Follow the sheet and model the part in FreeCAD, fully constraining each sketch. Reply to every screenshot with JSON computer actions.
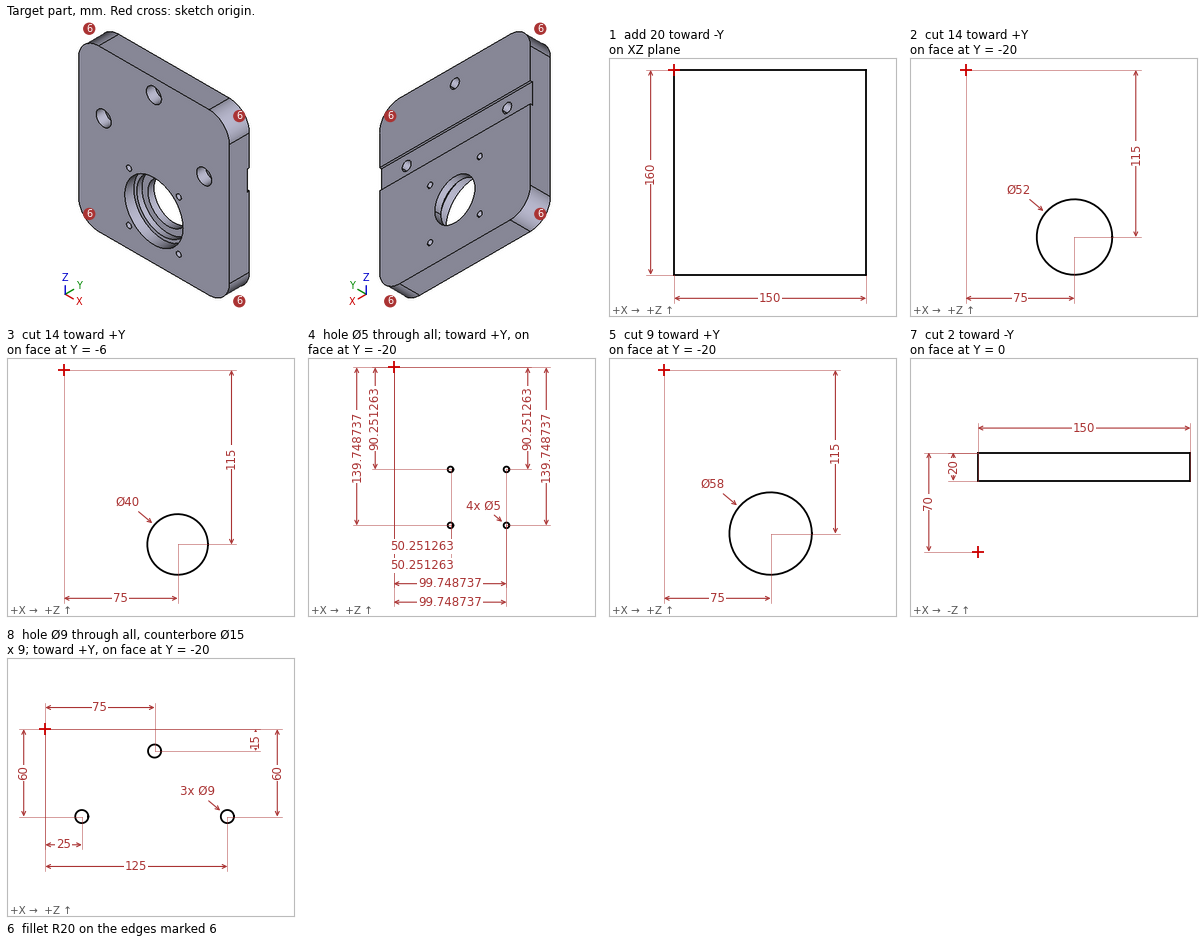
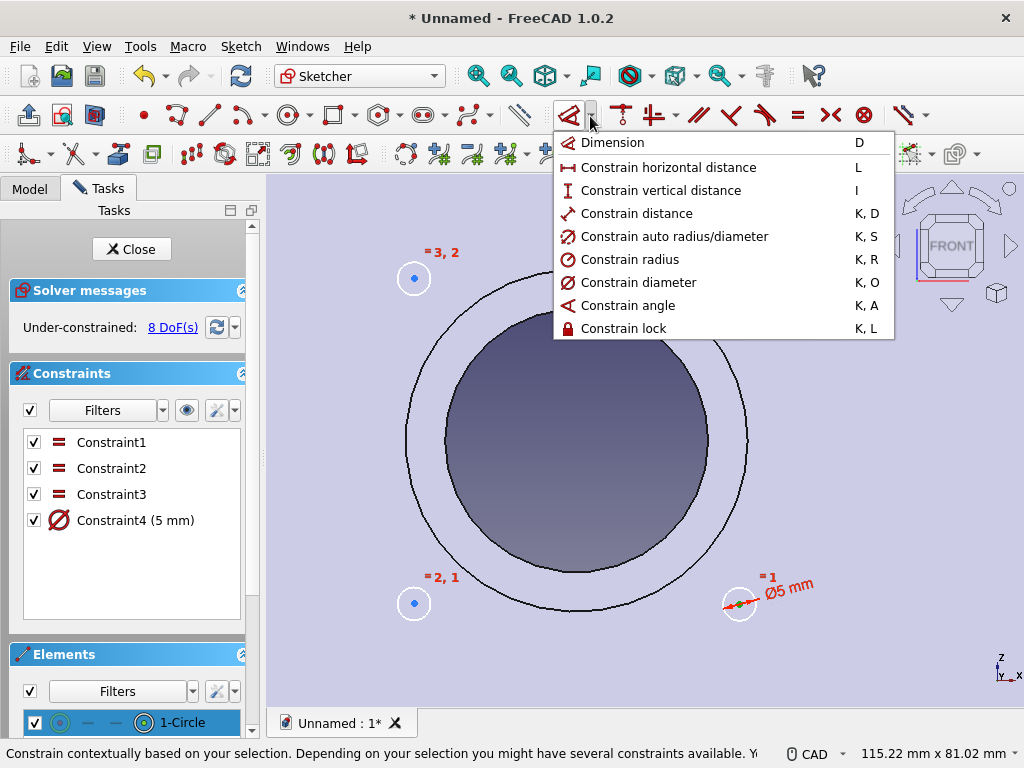
{"action": "left_click", "coordinate": [724, 168]}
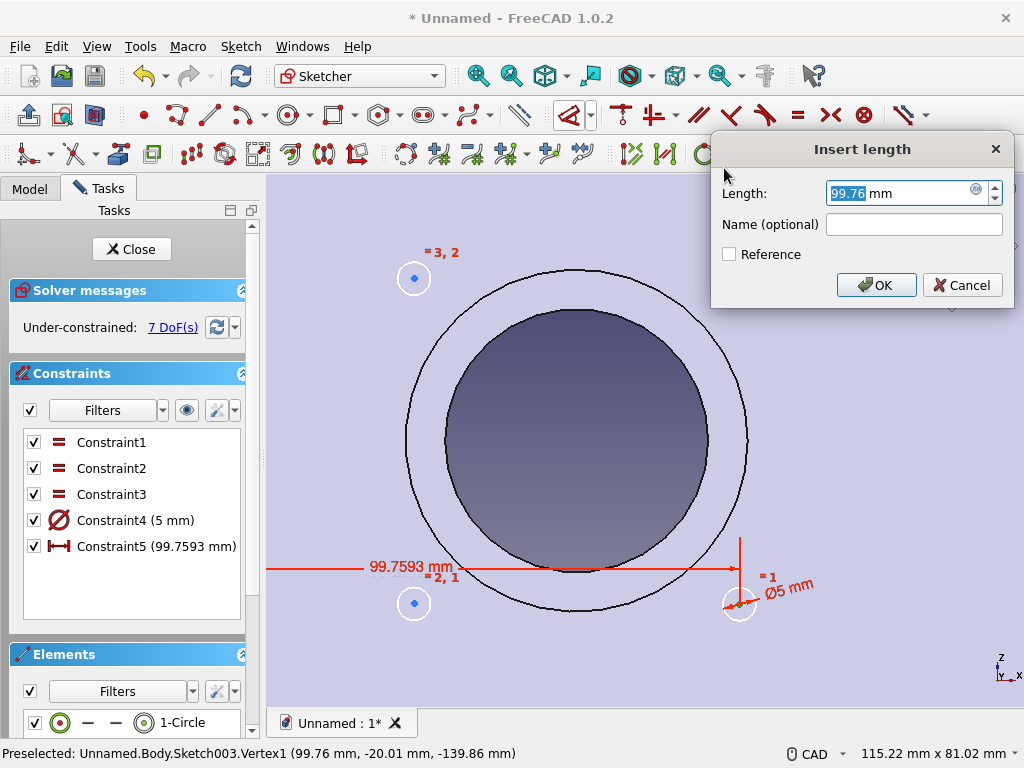
{"action": "type", "text": "99.748737"}
{"action": "key", "text": "Return"}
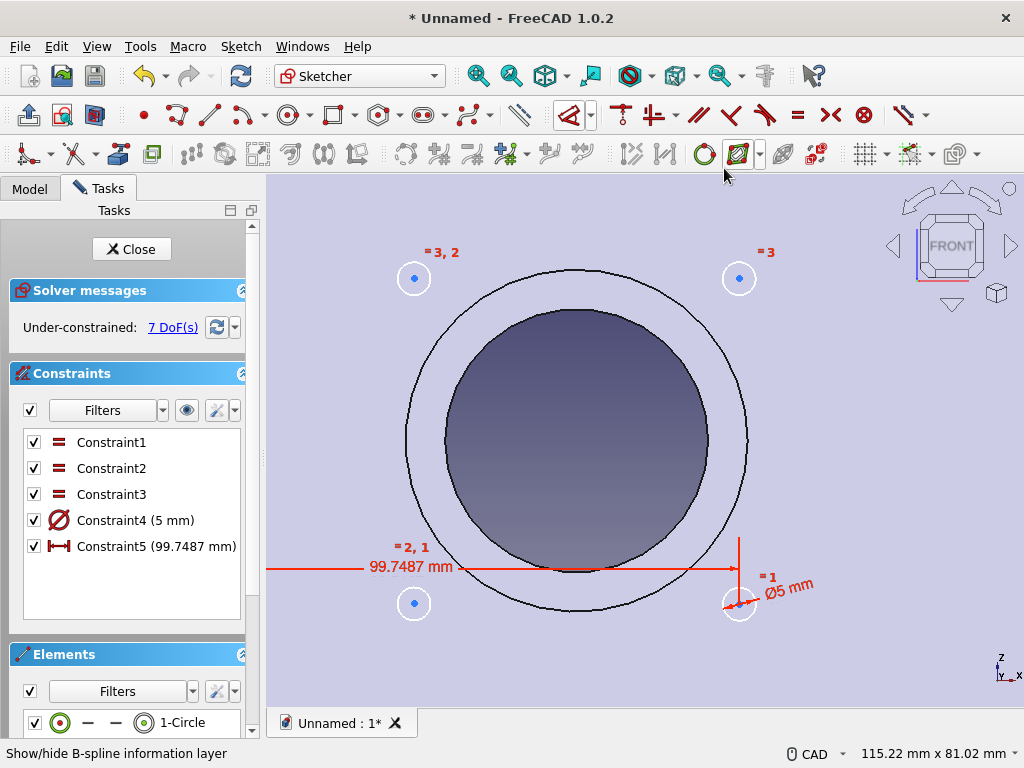
{"action": "left_click", "coordinate": [414, 604]}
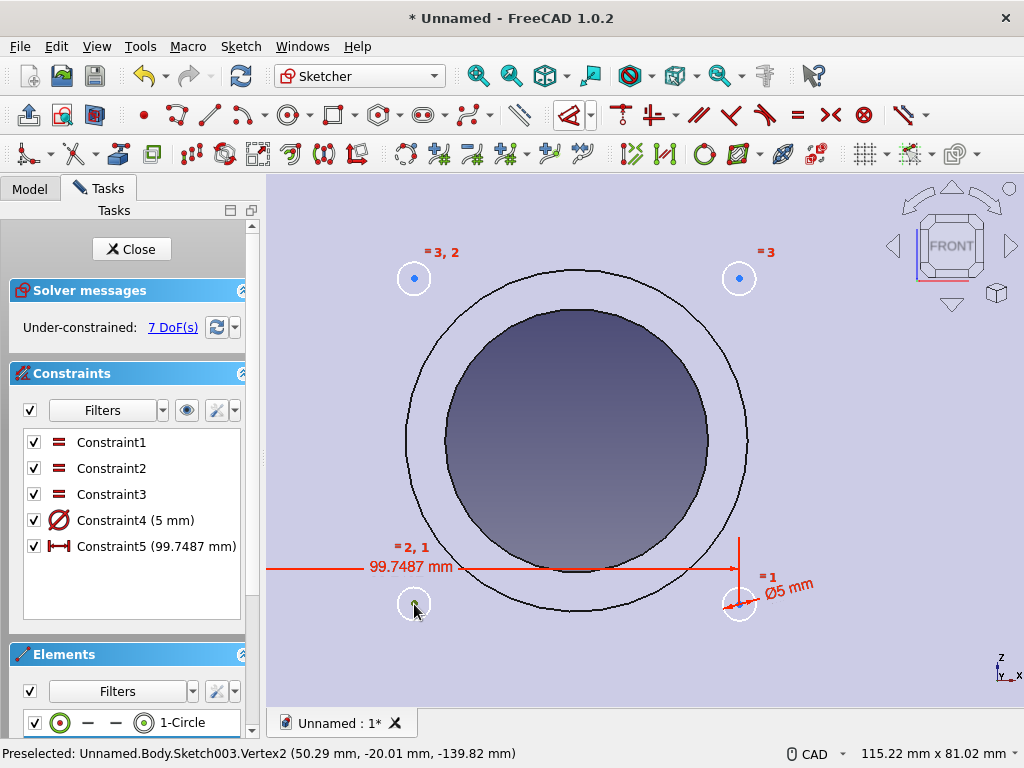
{"action": "key", "text": "l"}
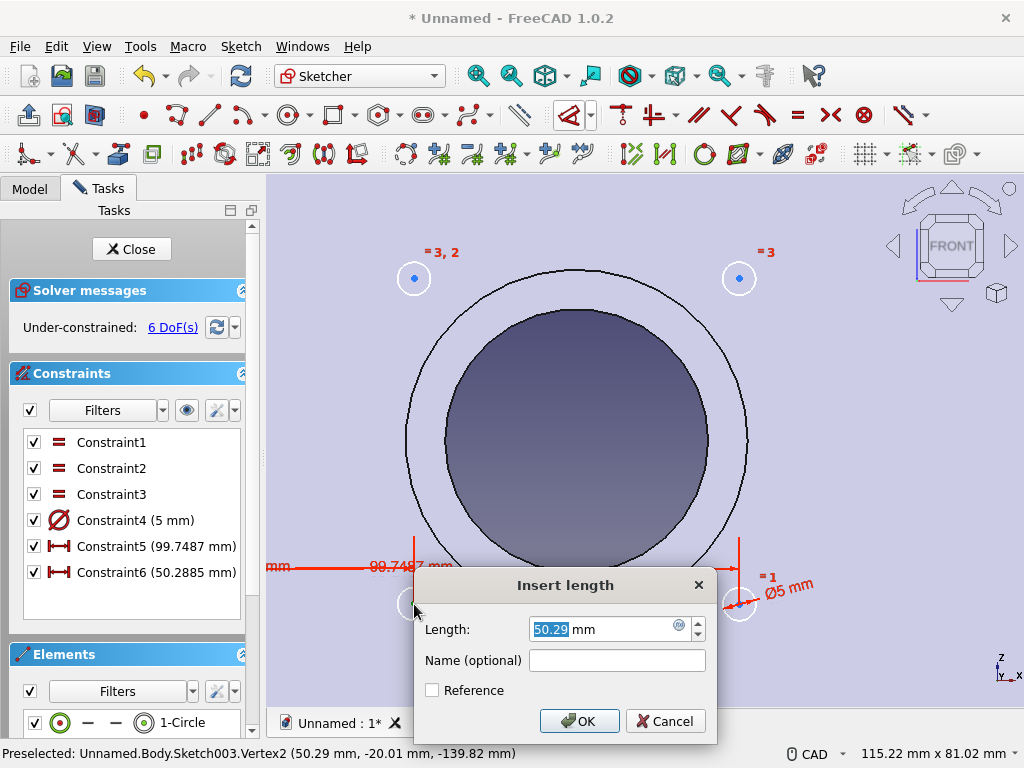
{"action": "type", "text": "50.251263"}
{"action": "key", "text": "Return"}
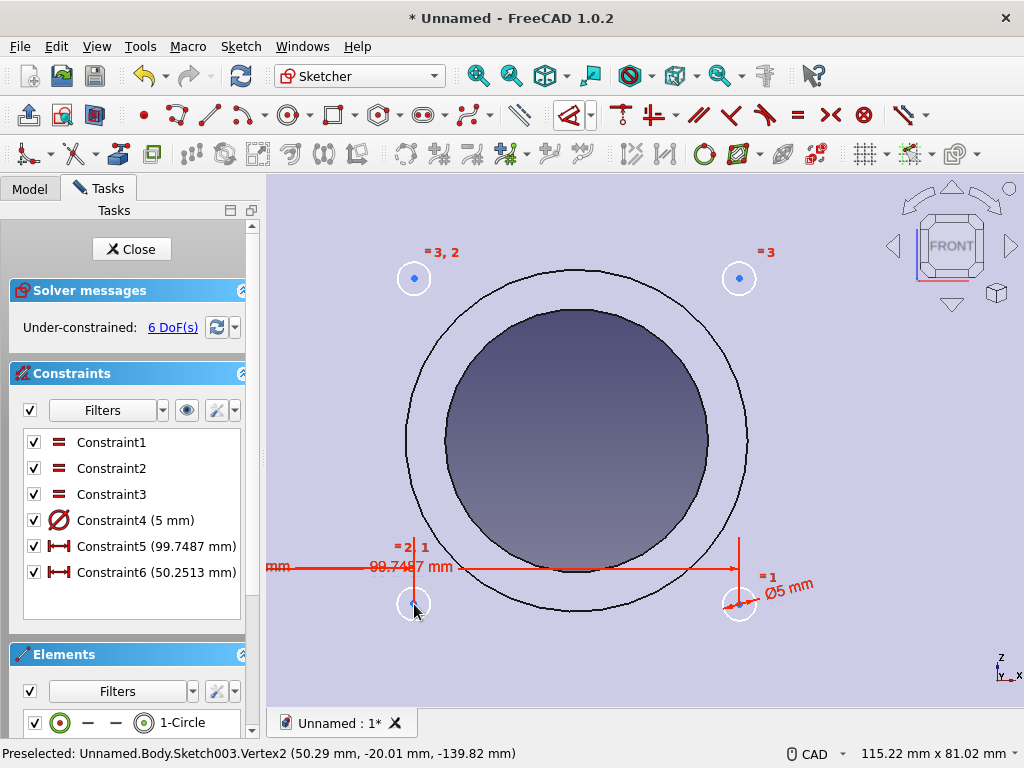
{"action": "left_click", "coordinate": [414, 279]}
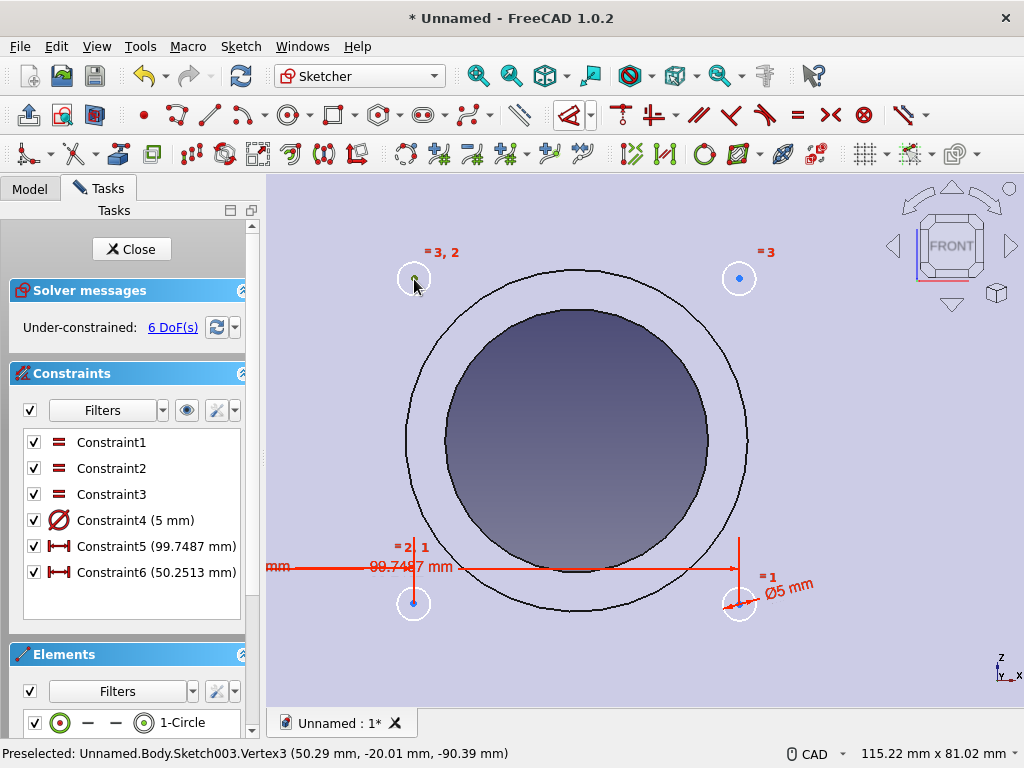
{"action": "key", "text": "l"}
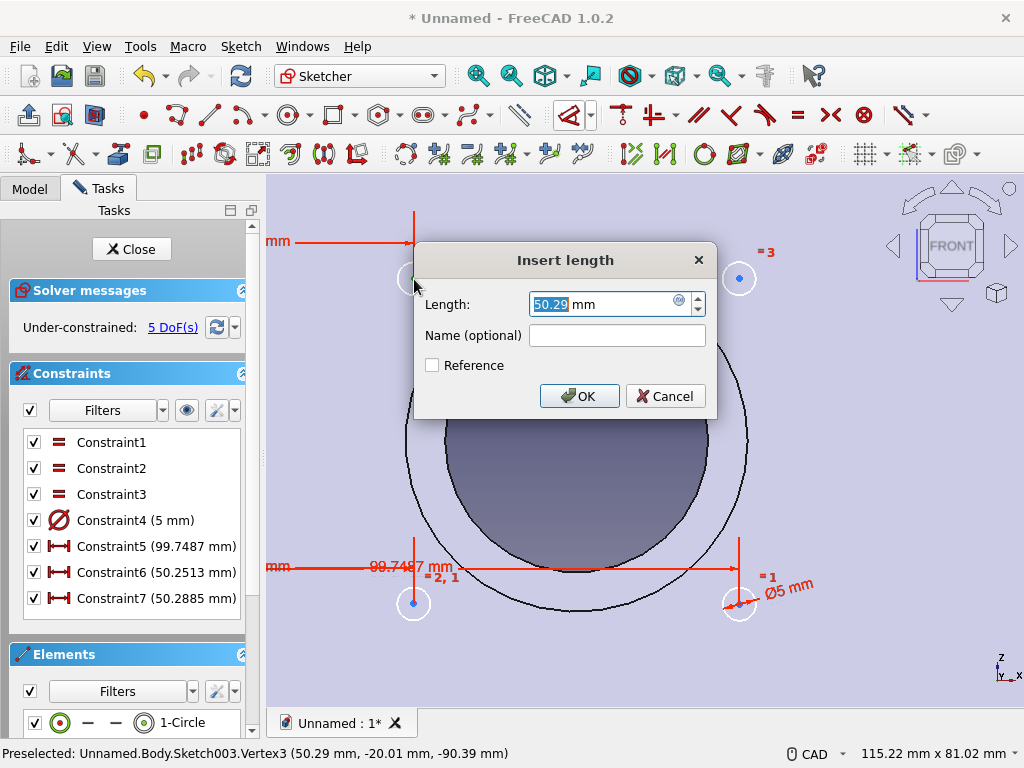
{"action": "type", "text": "50.251263"}
{"action": "key", "text": "Return"}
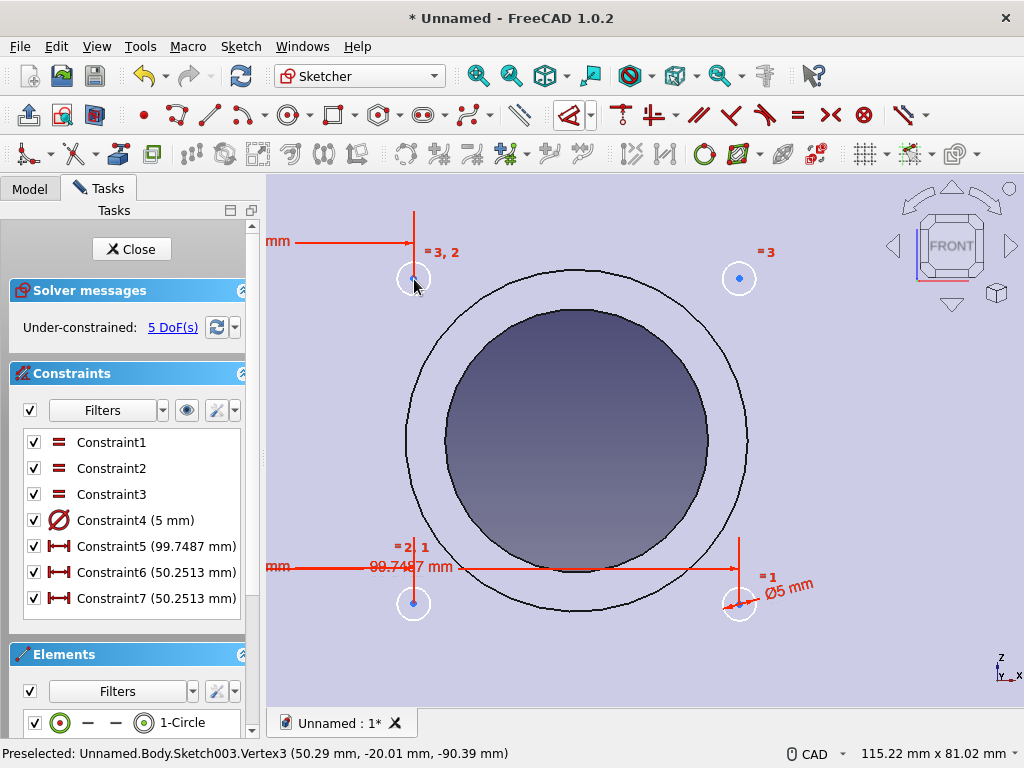
{"action": "left_click", "coordinate": [414, 279]}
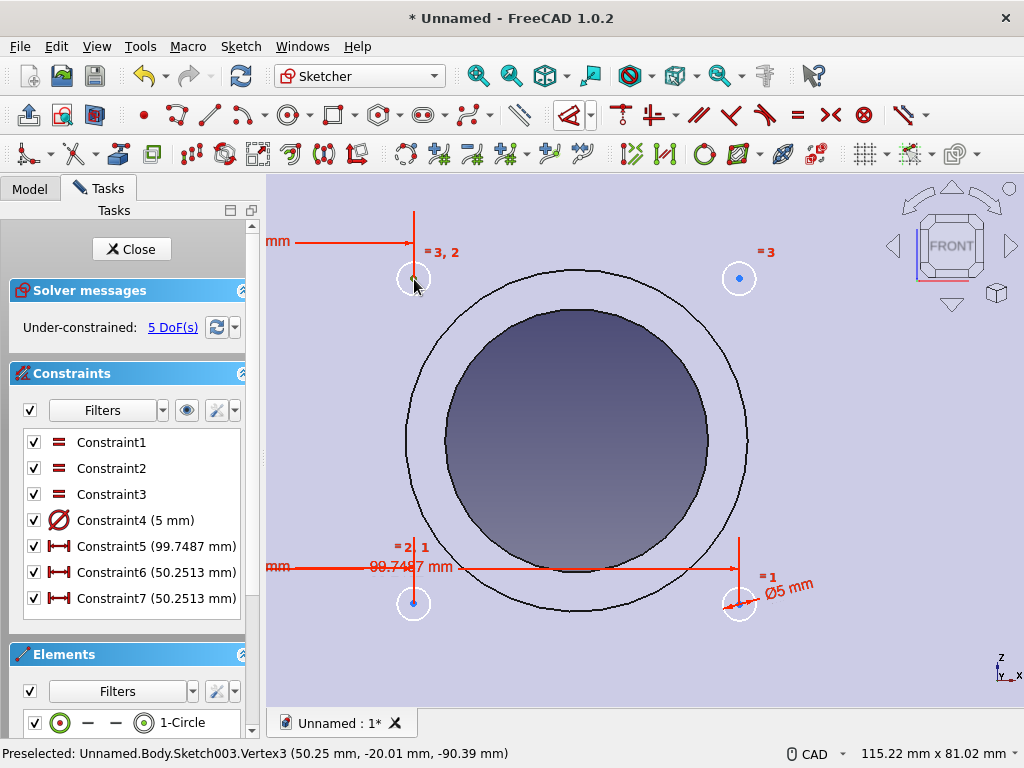
{"action": "left_click", "coordinate": [590, 116]}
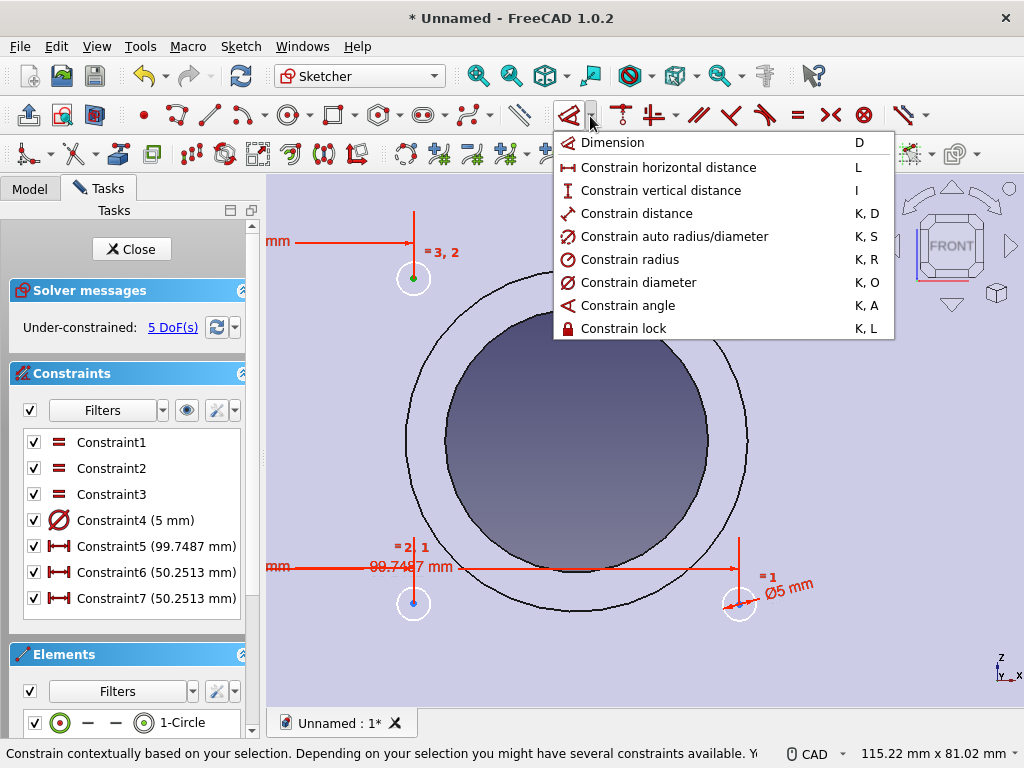
{"action": "left_click", "coordinate": [724, 190]}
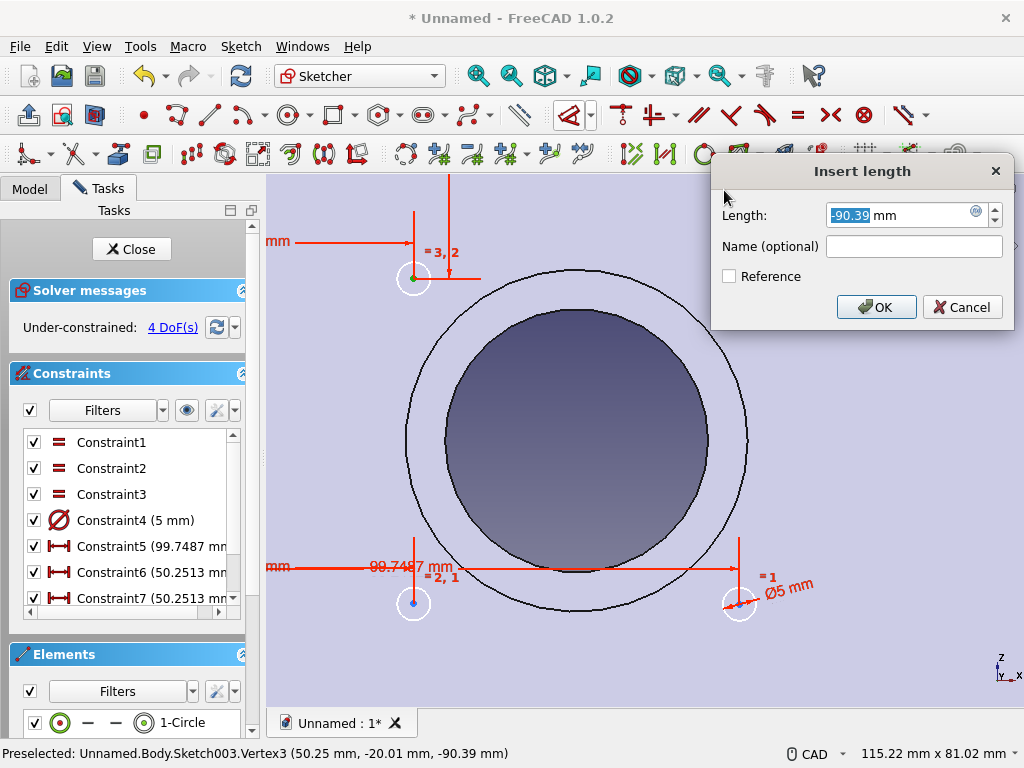
{"action": "type", "text": "-90.251263"}
{"action": "key", "text": "Return"}